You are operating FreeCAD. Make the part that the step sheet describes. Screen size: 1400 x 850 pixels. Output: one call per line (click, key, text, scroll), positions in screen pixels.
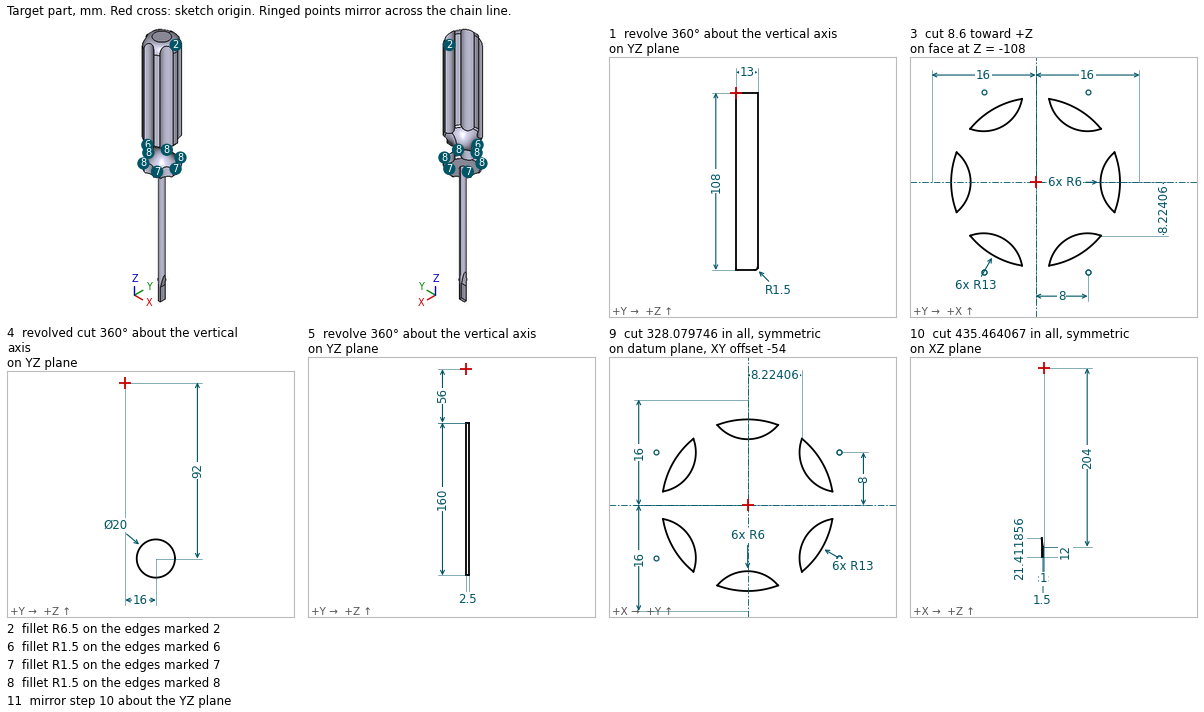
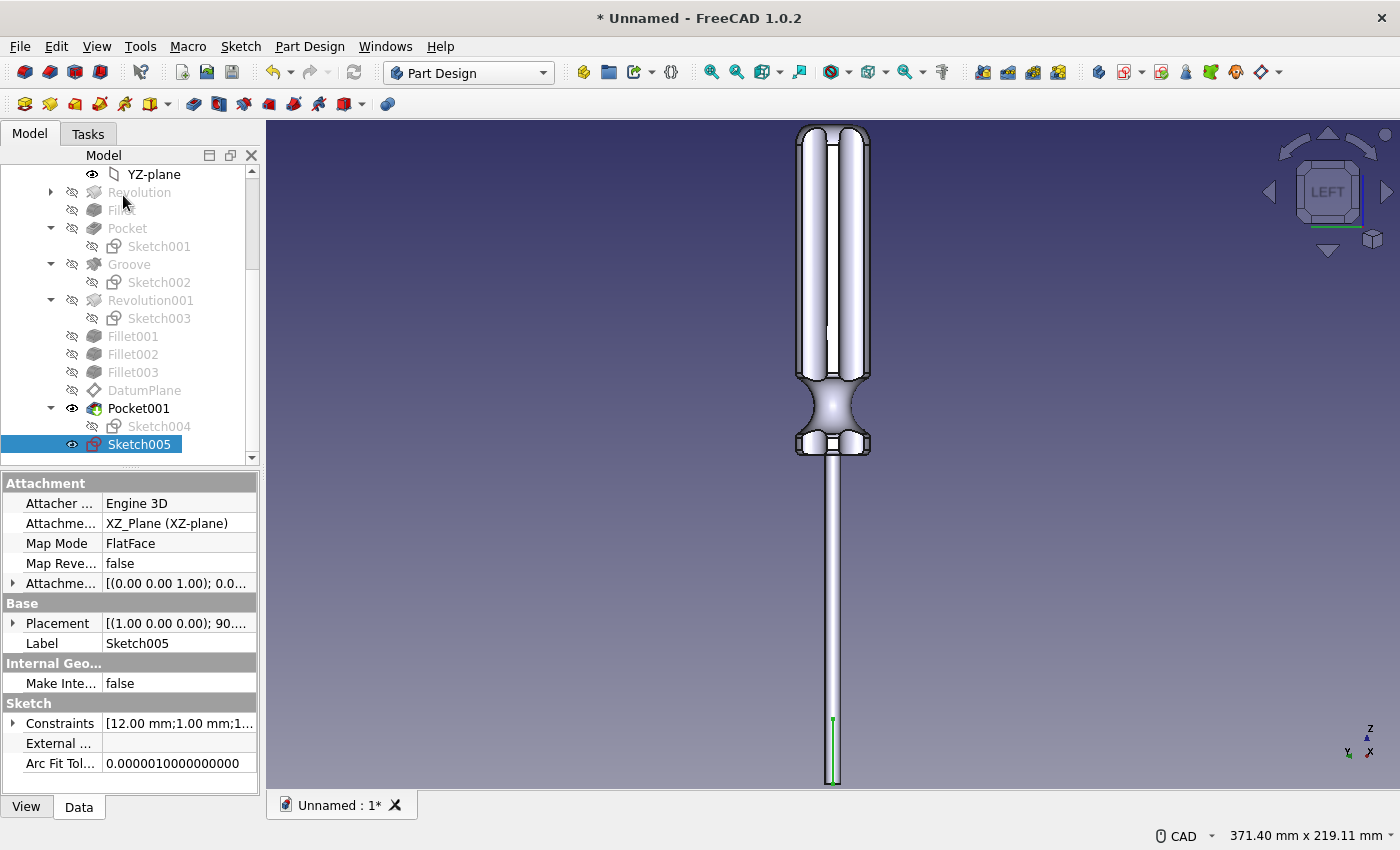
click(194, 104)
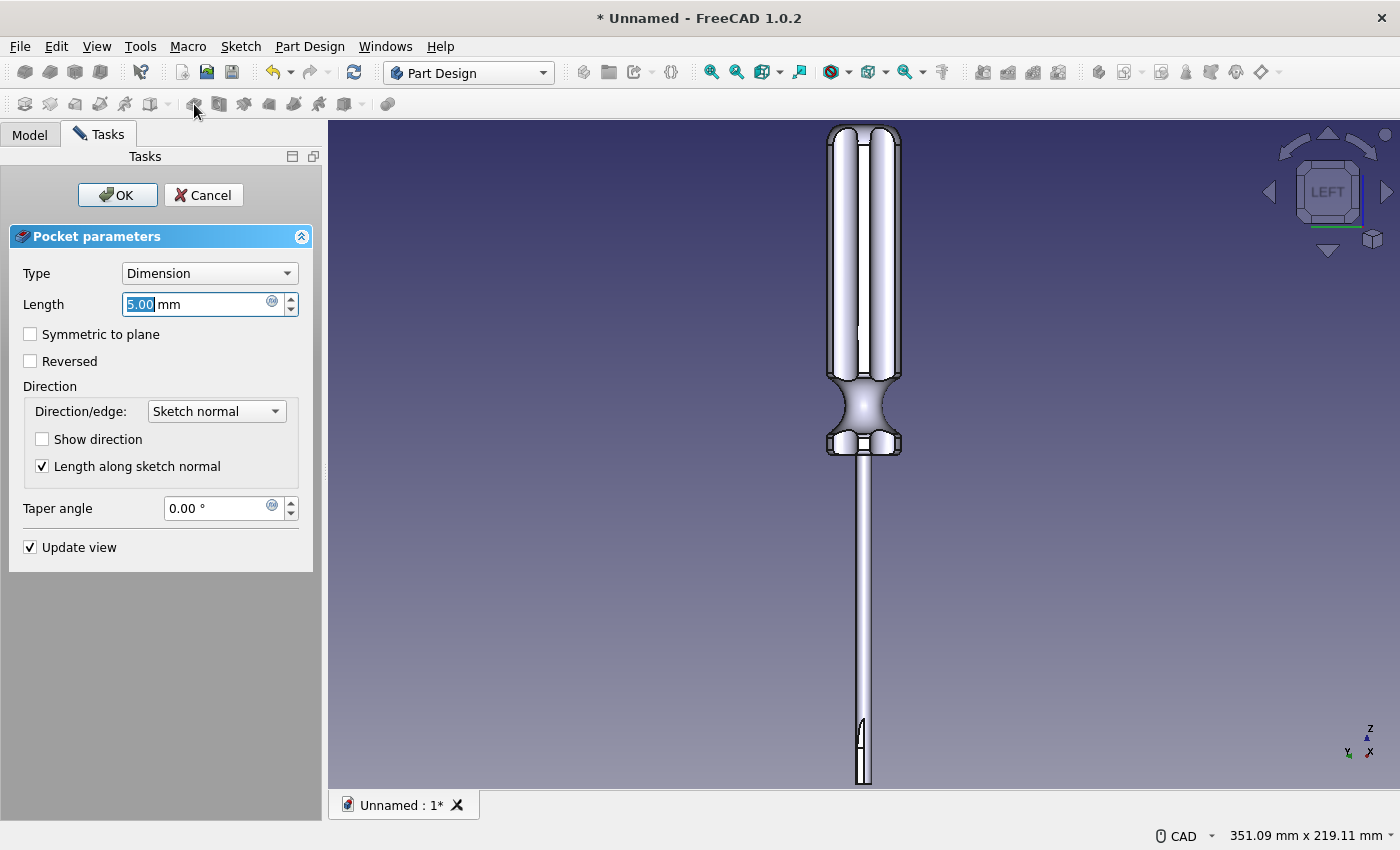
text(435.464067)
key(Tab)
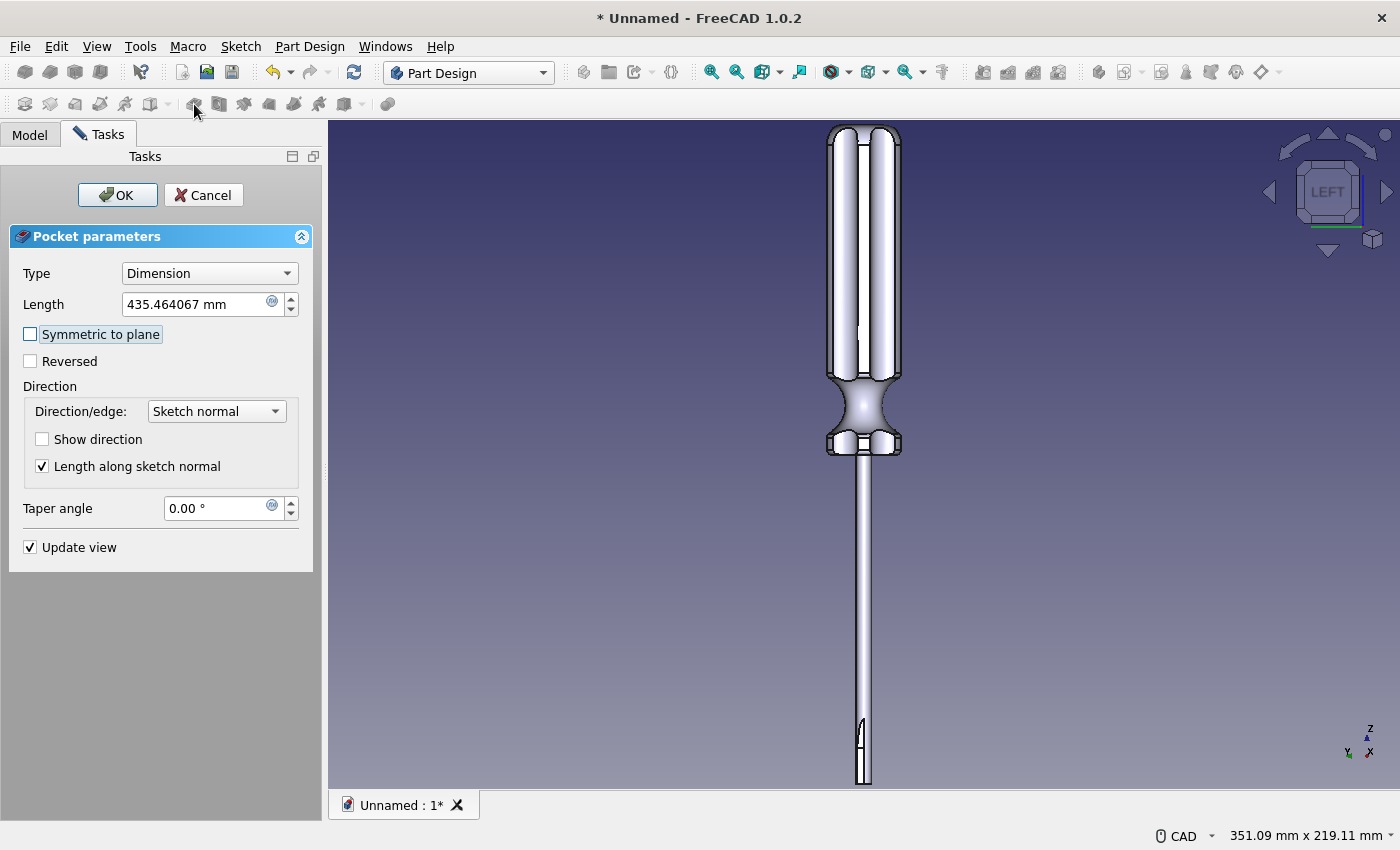
click(31, 334)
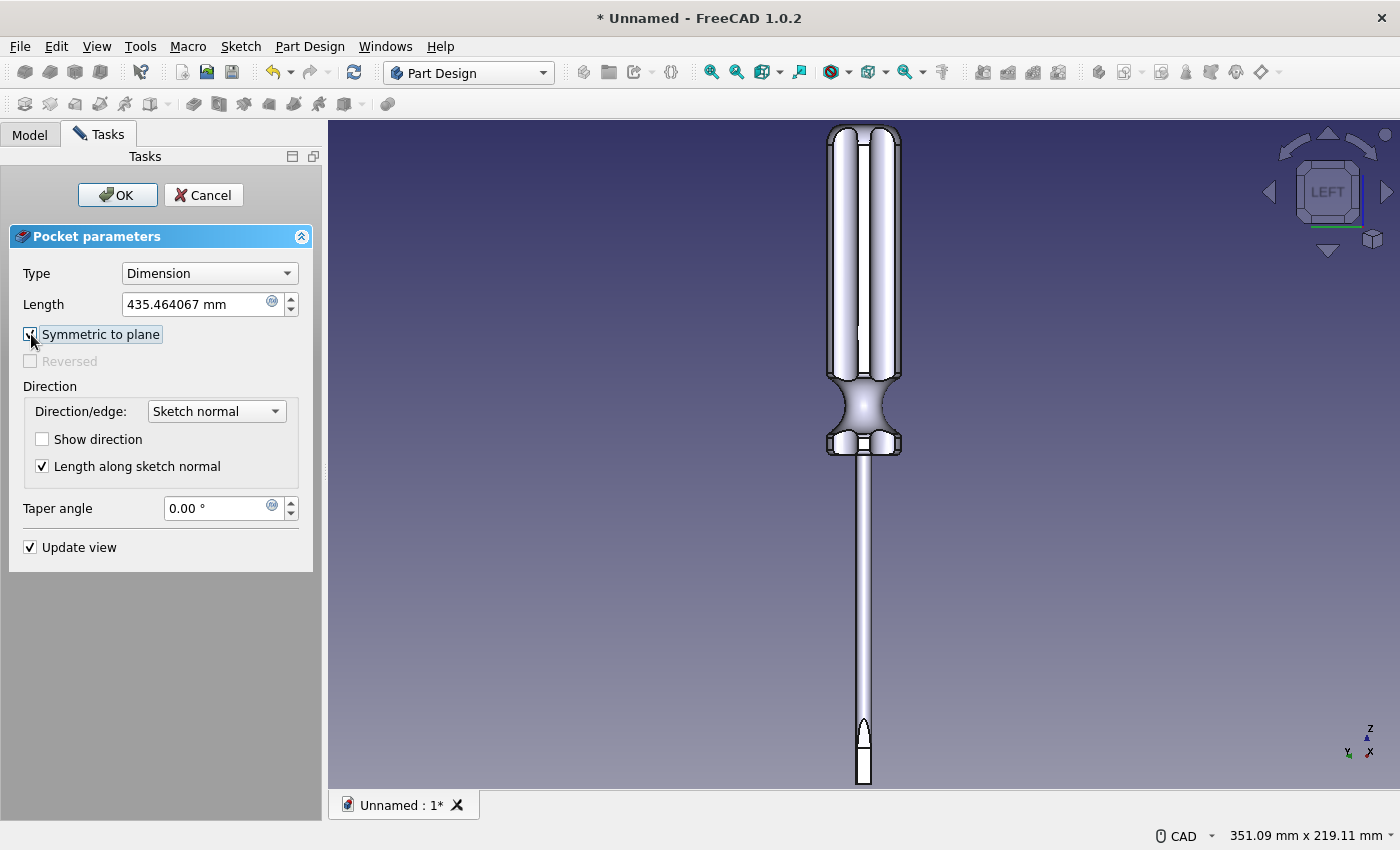
click(118, 195)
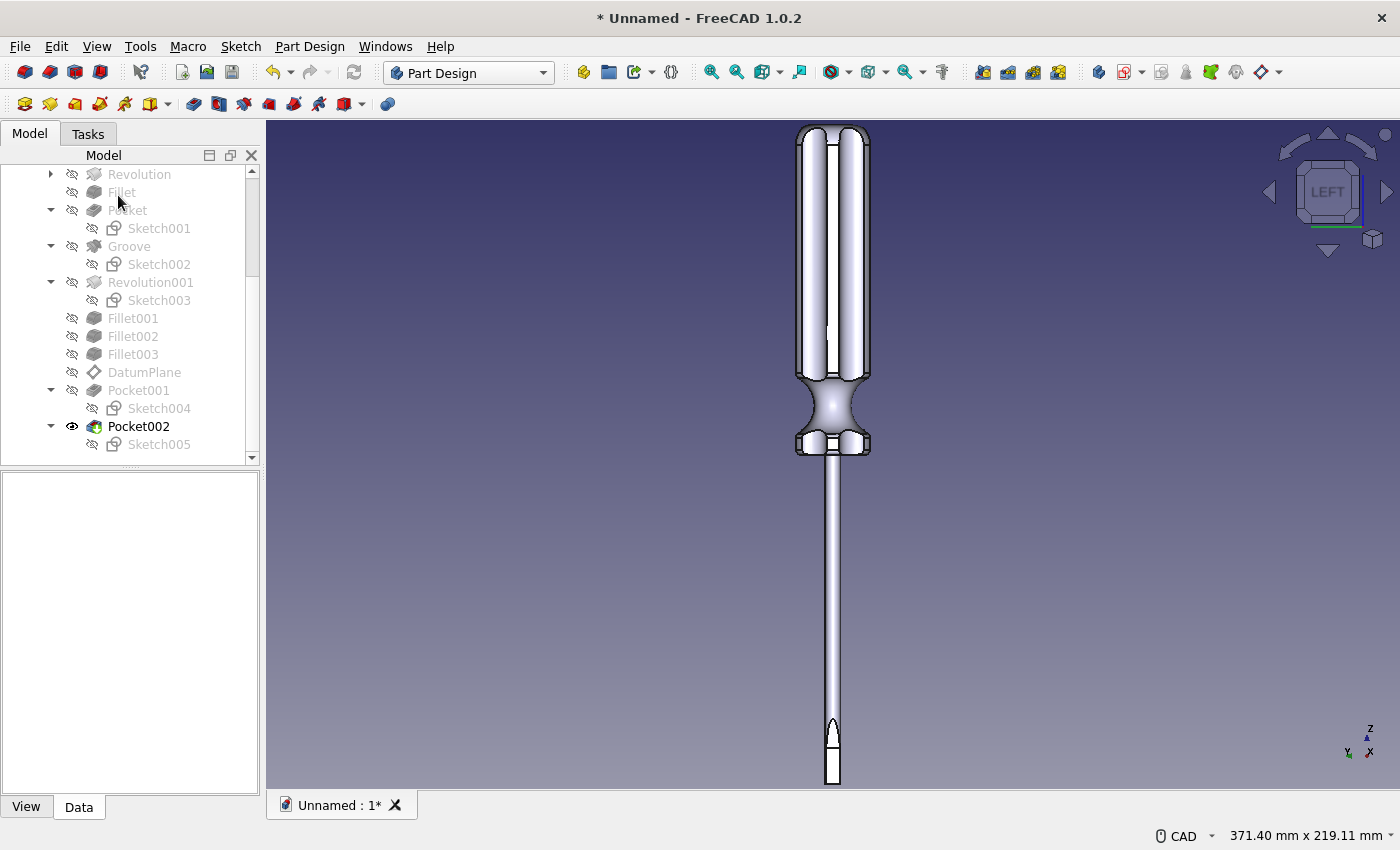
click(117, 426)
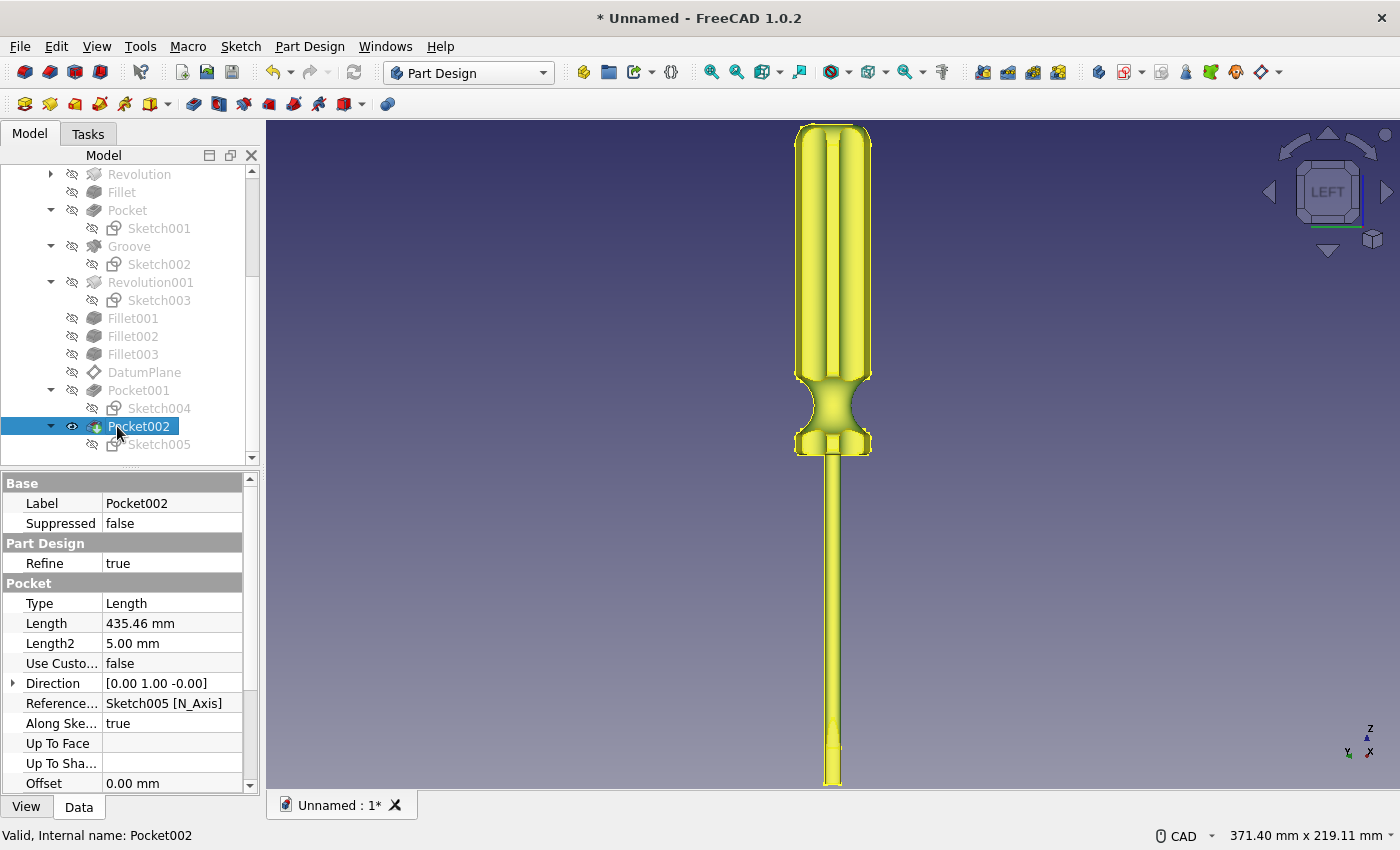
click(983, 72)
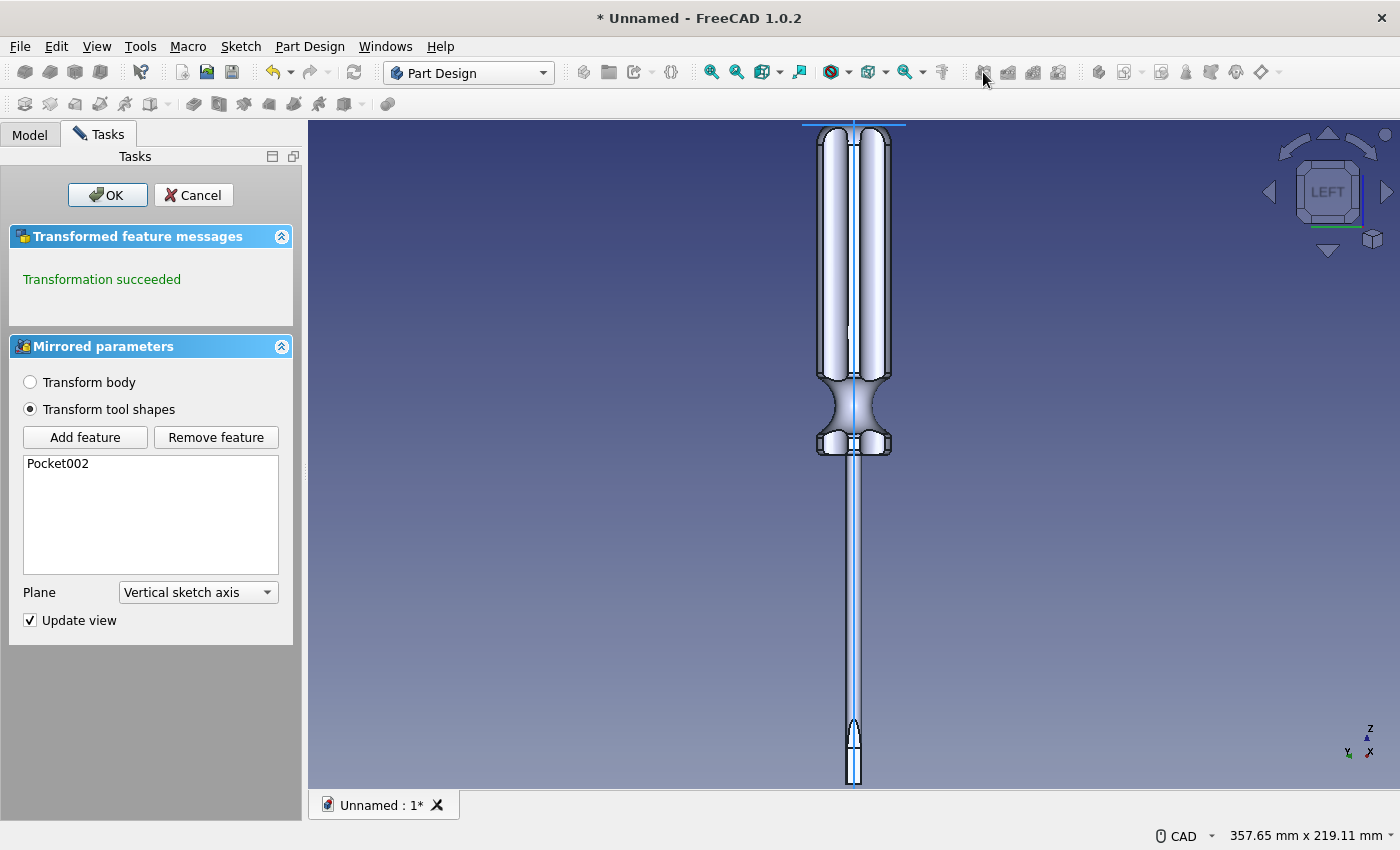
click(199, 592)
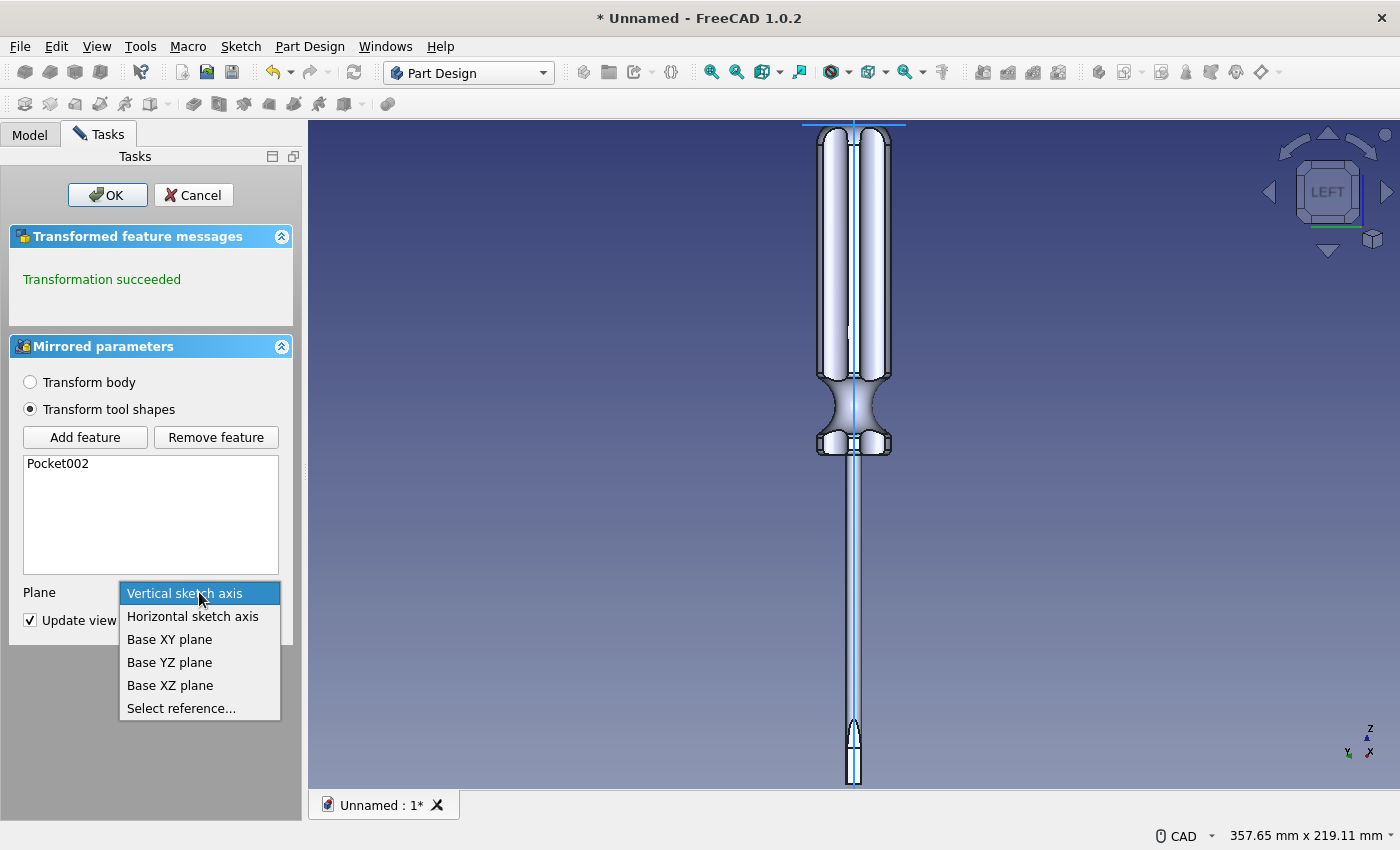
click(198, 662)